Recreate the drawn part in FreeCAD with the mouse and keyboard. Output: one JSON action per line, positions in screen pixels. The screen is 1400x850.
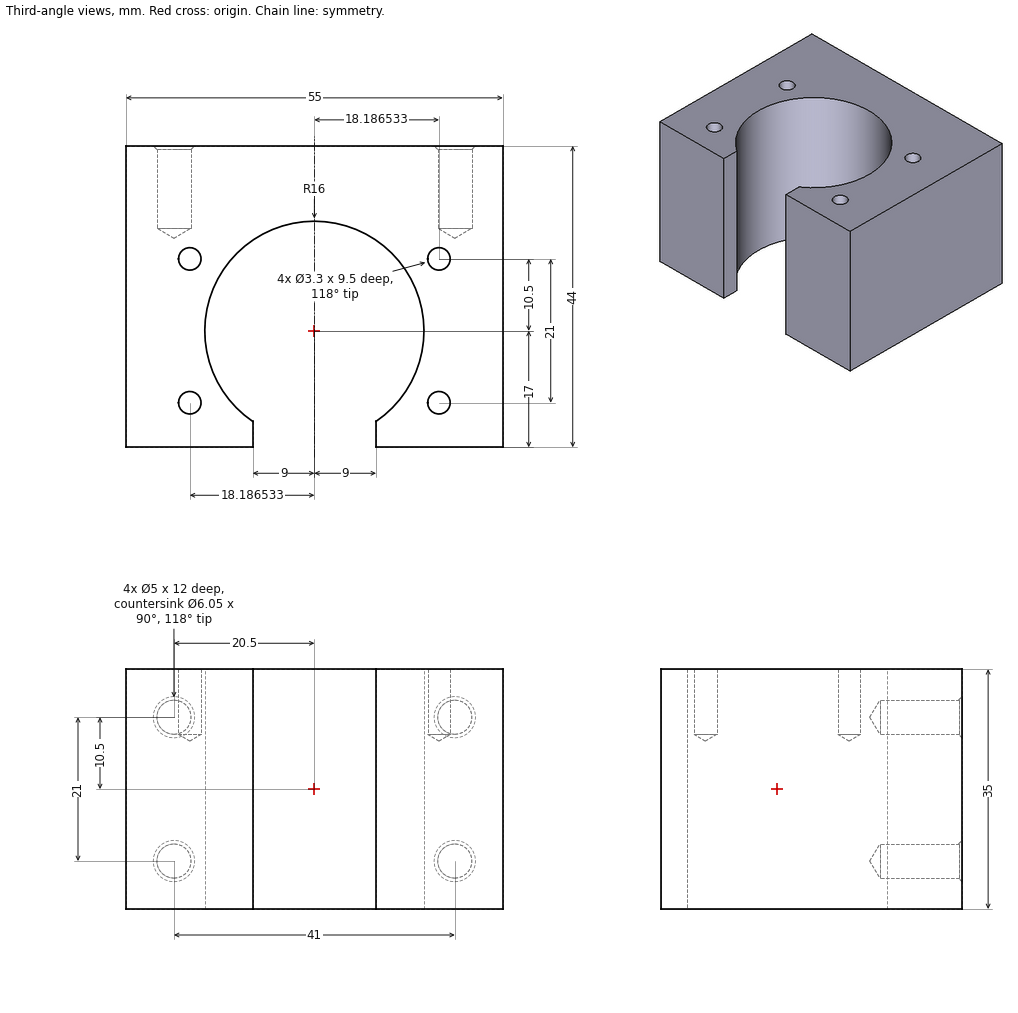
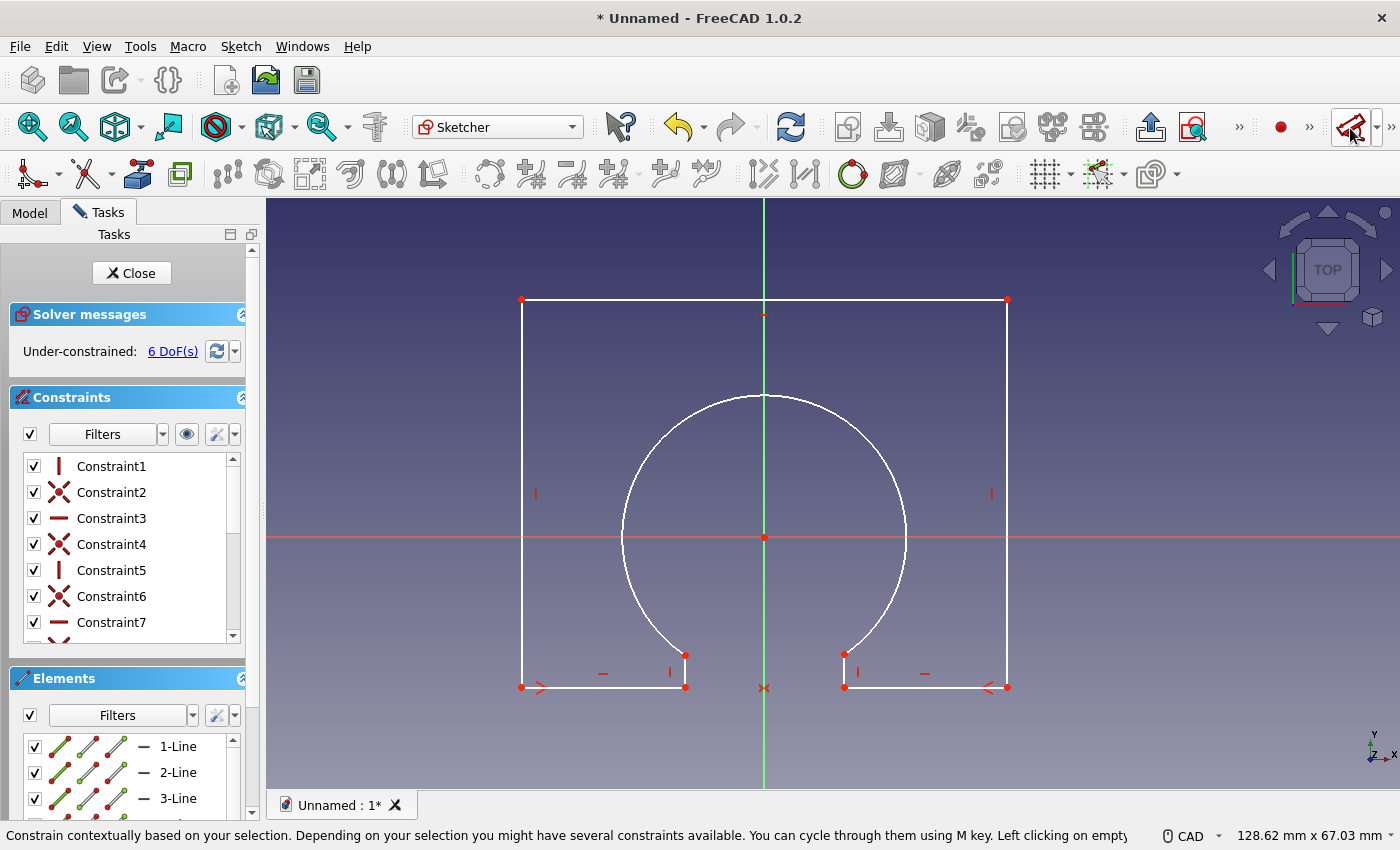
{"action": "left_click", "coordinate": [885, 463]}
{"action": "left_click", "coordinate": [912, 446]}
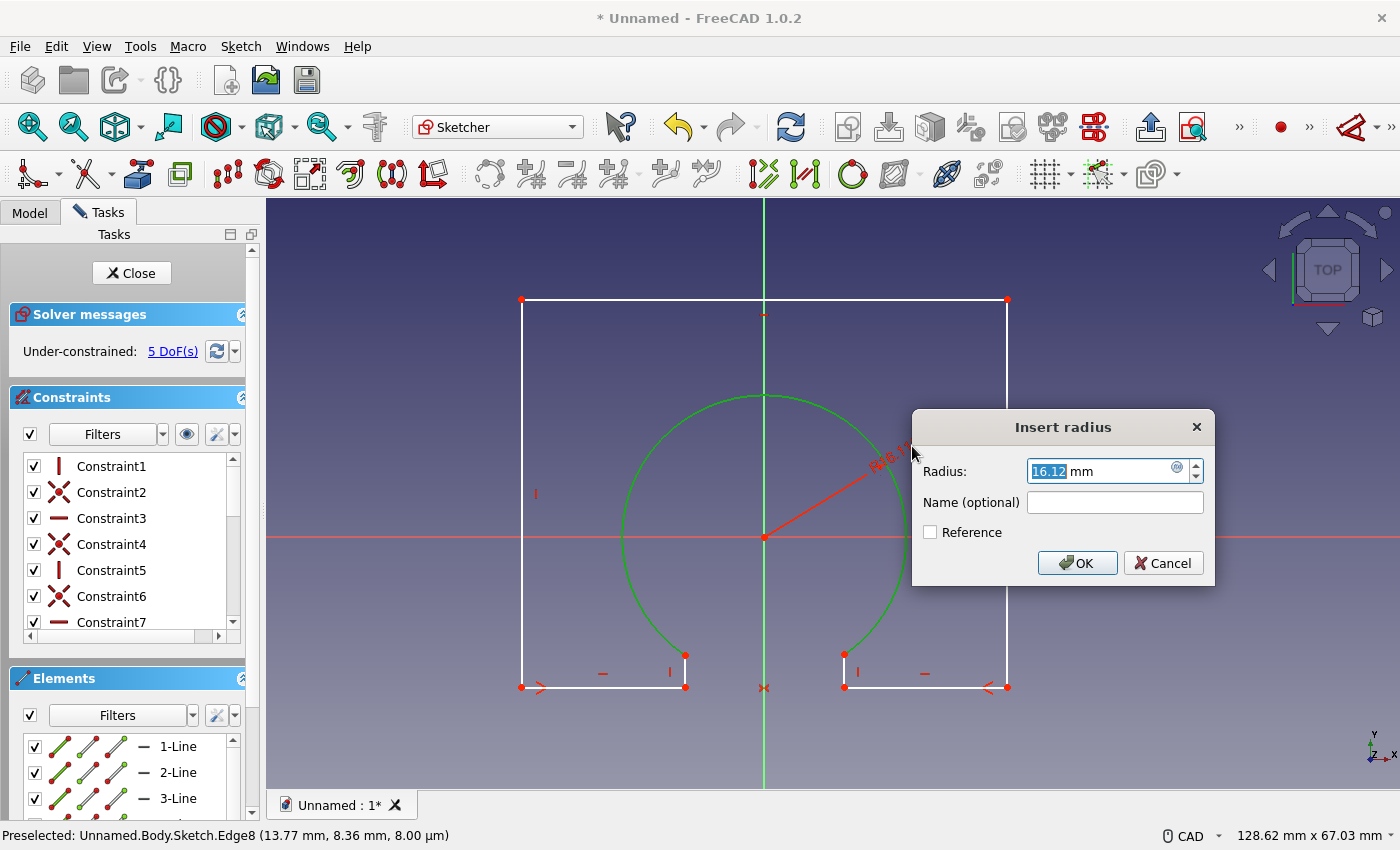
{"action": "type", "text": "16"}
{"action": "key", "text": "Return"}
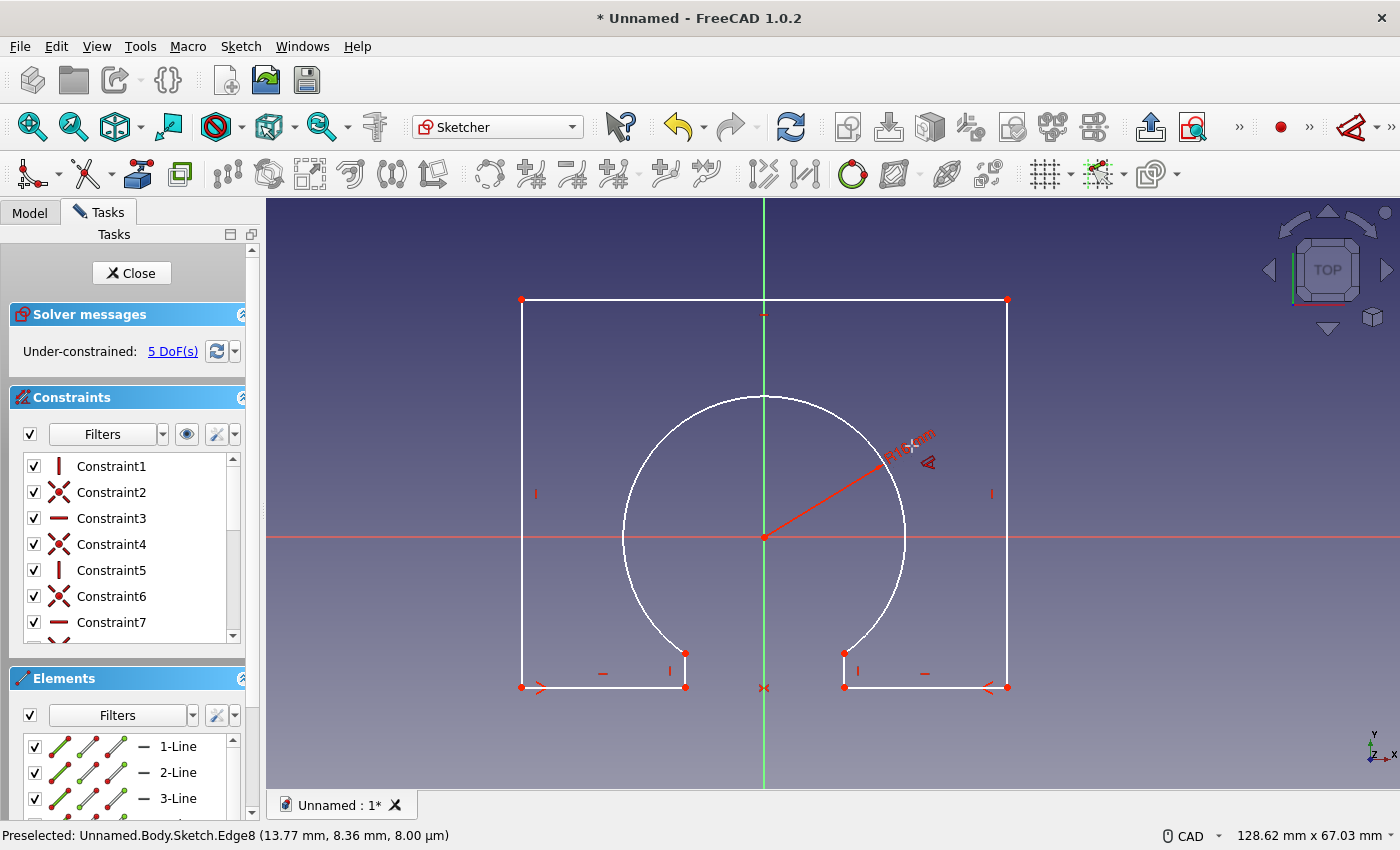
{"action": "left_click", "coordinate": [1007, 572]}
{"action": "left_click", "coordinate": [1041, 494]}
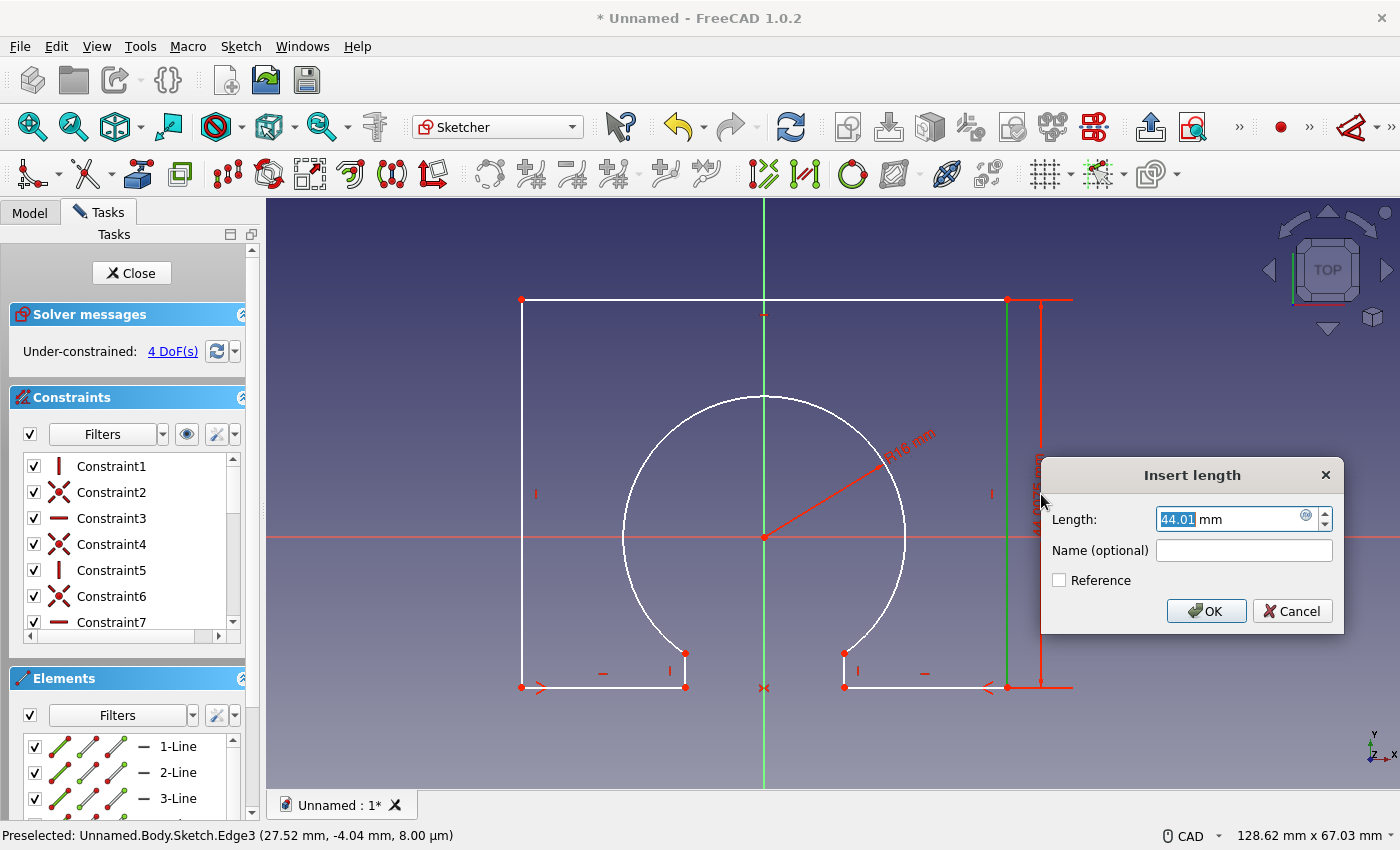
{"action": "type", "text": "44"}
{"action": "key", "text": "Return"}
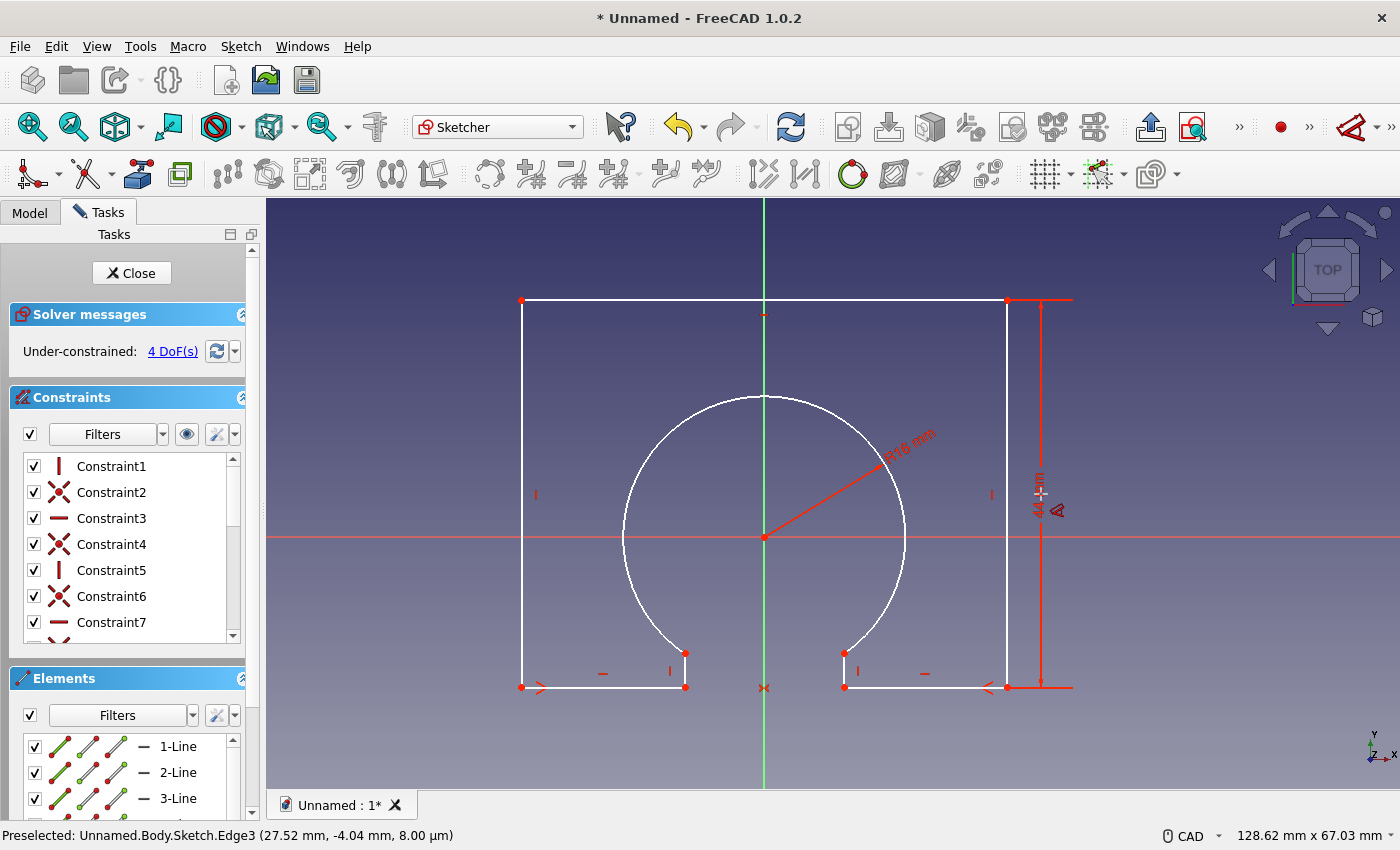
{"action": "left_click", "coordinate": [861, 300]}
{"action": "left_click", "coordinate": [653, 266]}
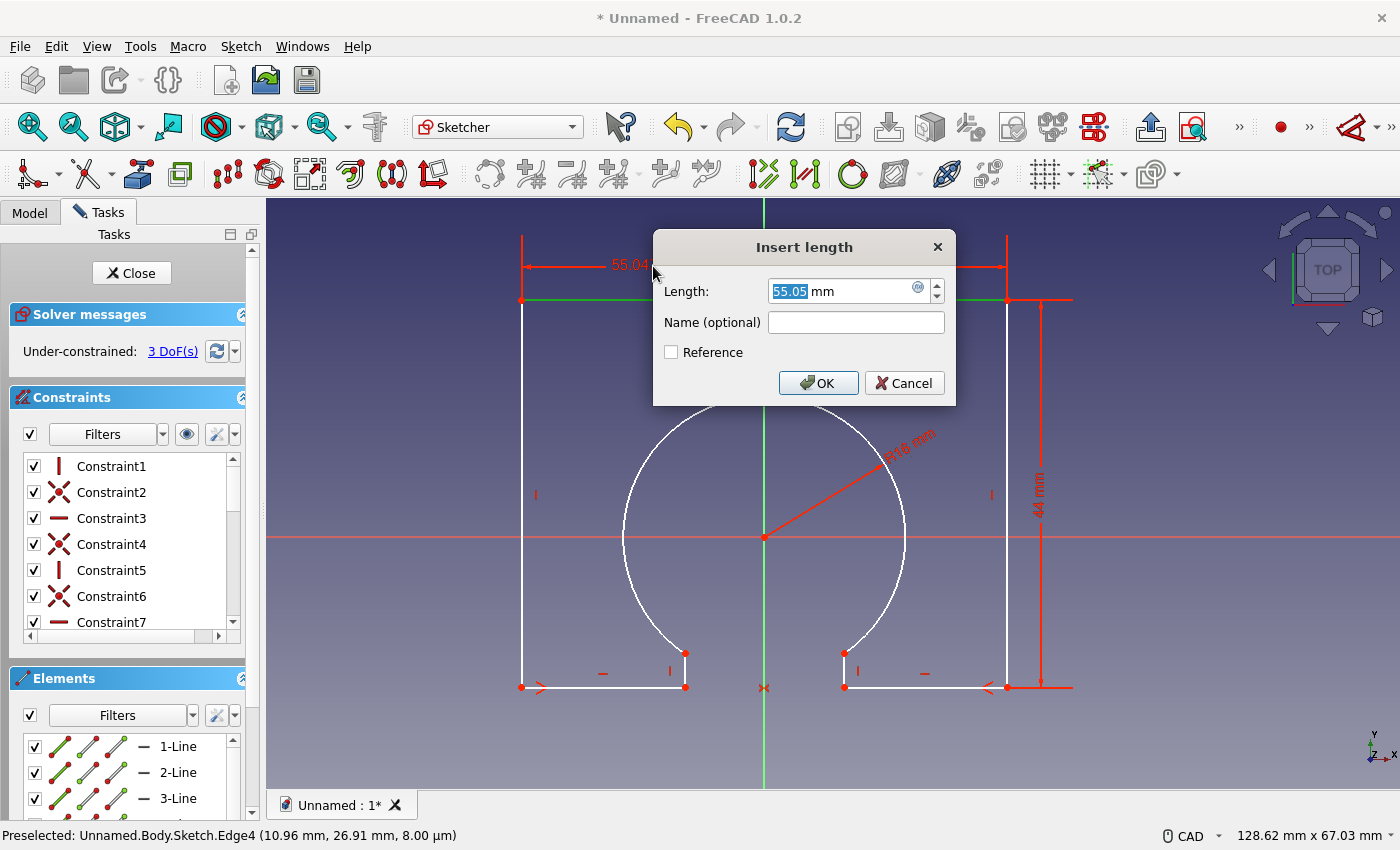
{"action": "type", "text": "55"}
{"action": "key", "text": "Return"}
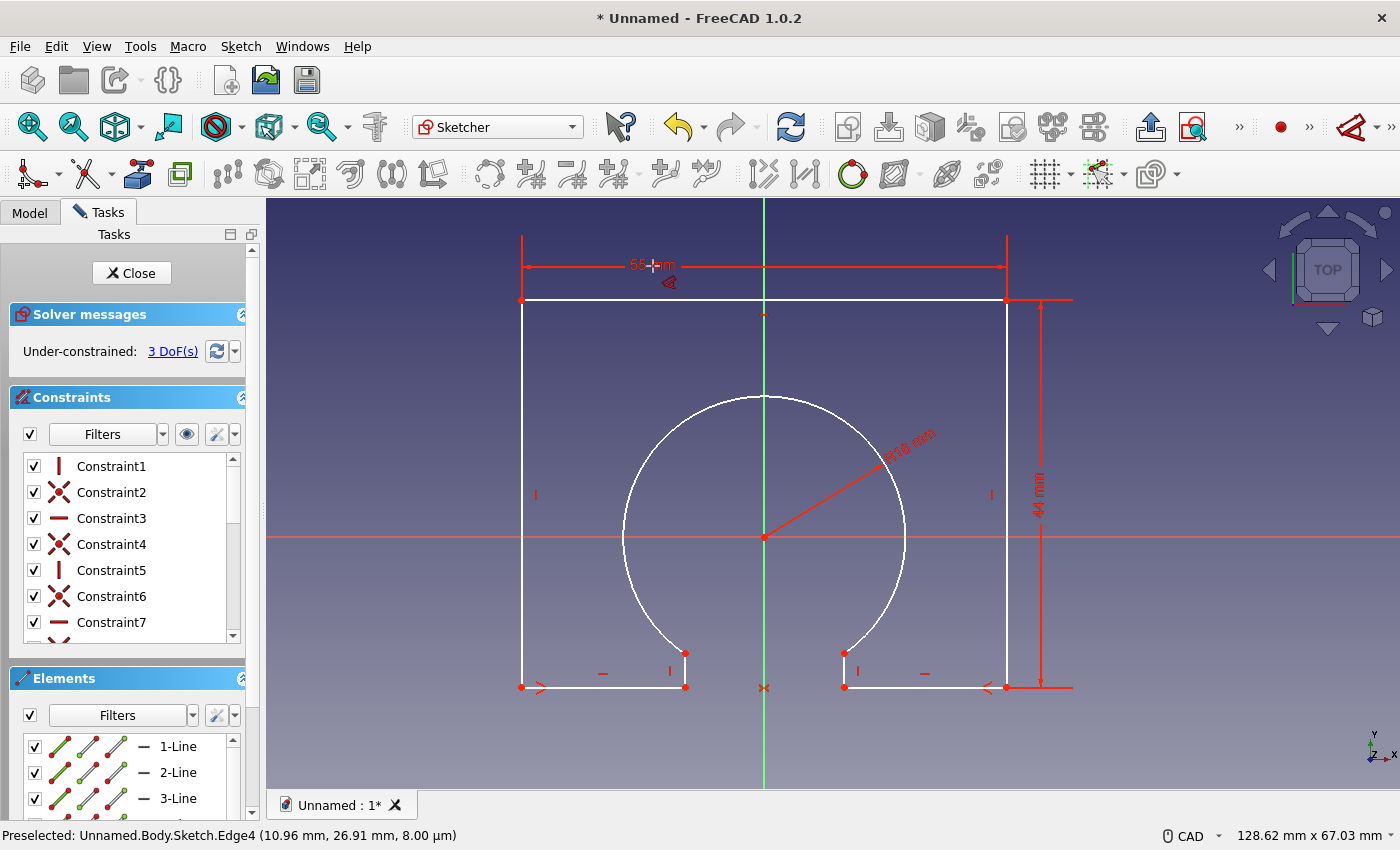
{"action": "left_click", "coordinate": [844, 654]}
{"action": "left_click", "coordinate": [804, 688]}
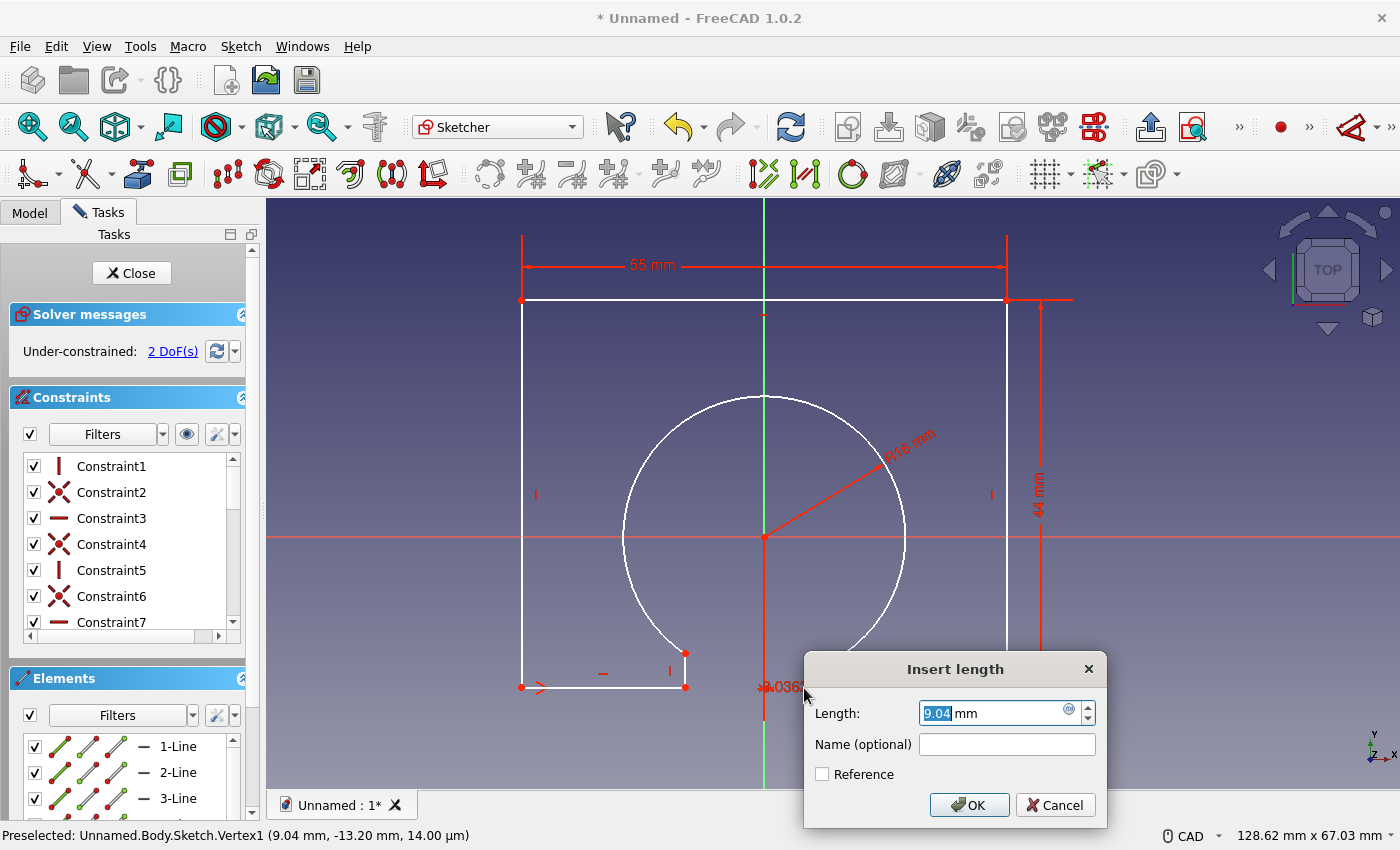
{"action": "type", "text": "9"}
{"action": "key", "text": "Return"}